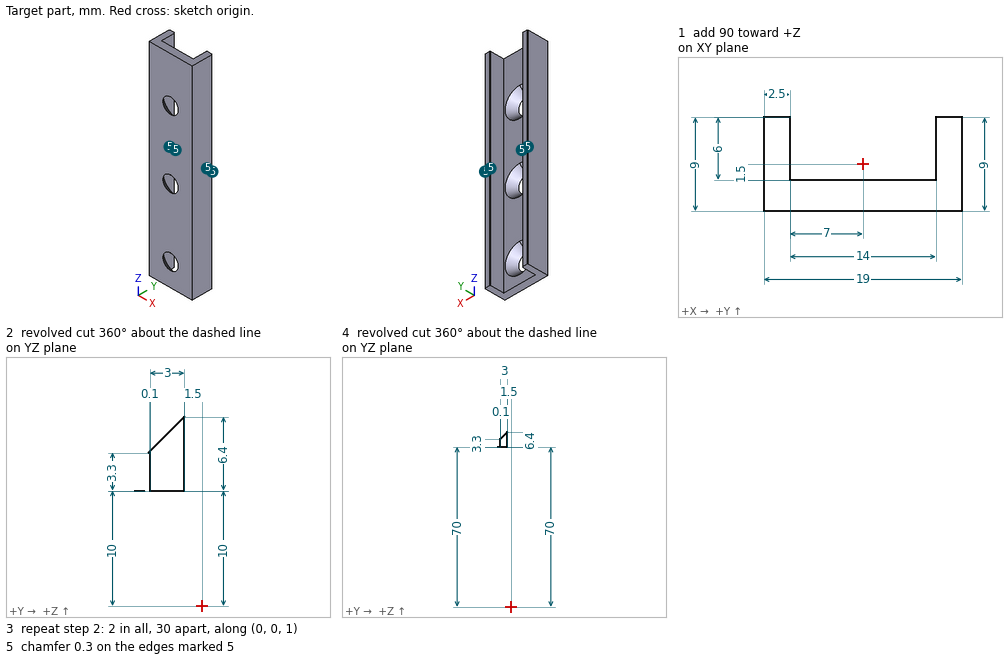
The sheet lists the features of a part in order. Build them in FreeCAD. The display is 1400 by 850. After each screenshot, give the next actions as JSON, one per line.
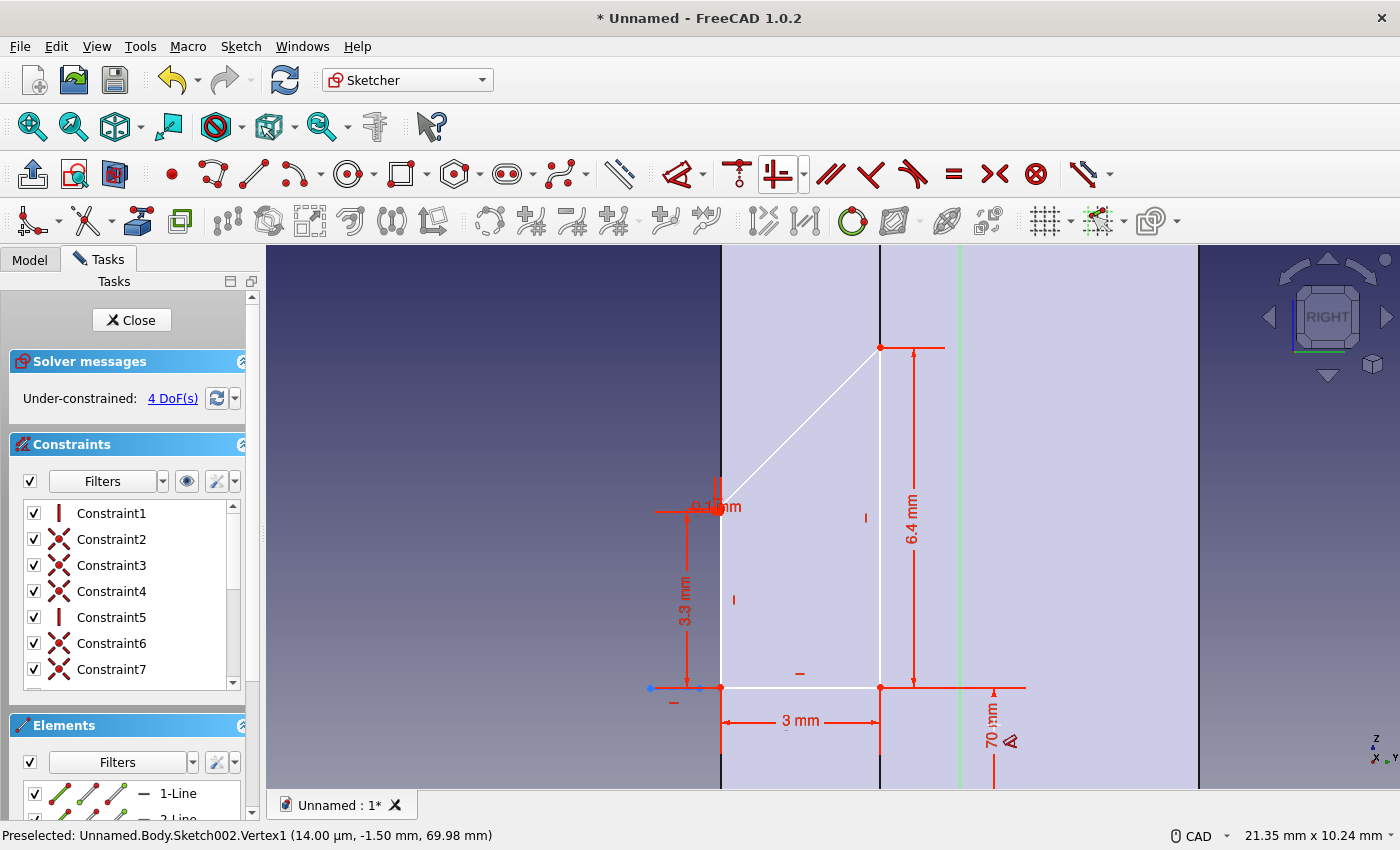
{"action": "left_click", "coordinate": [699, 689]}
{"action": "left_click", "coordinate": [994, 700]}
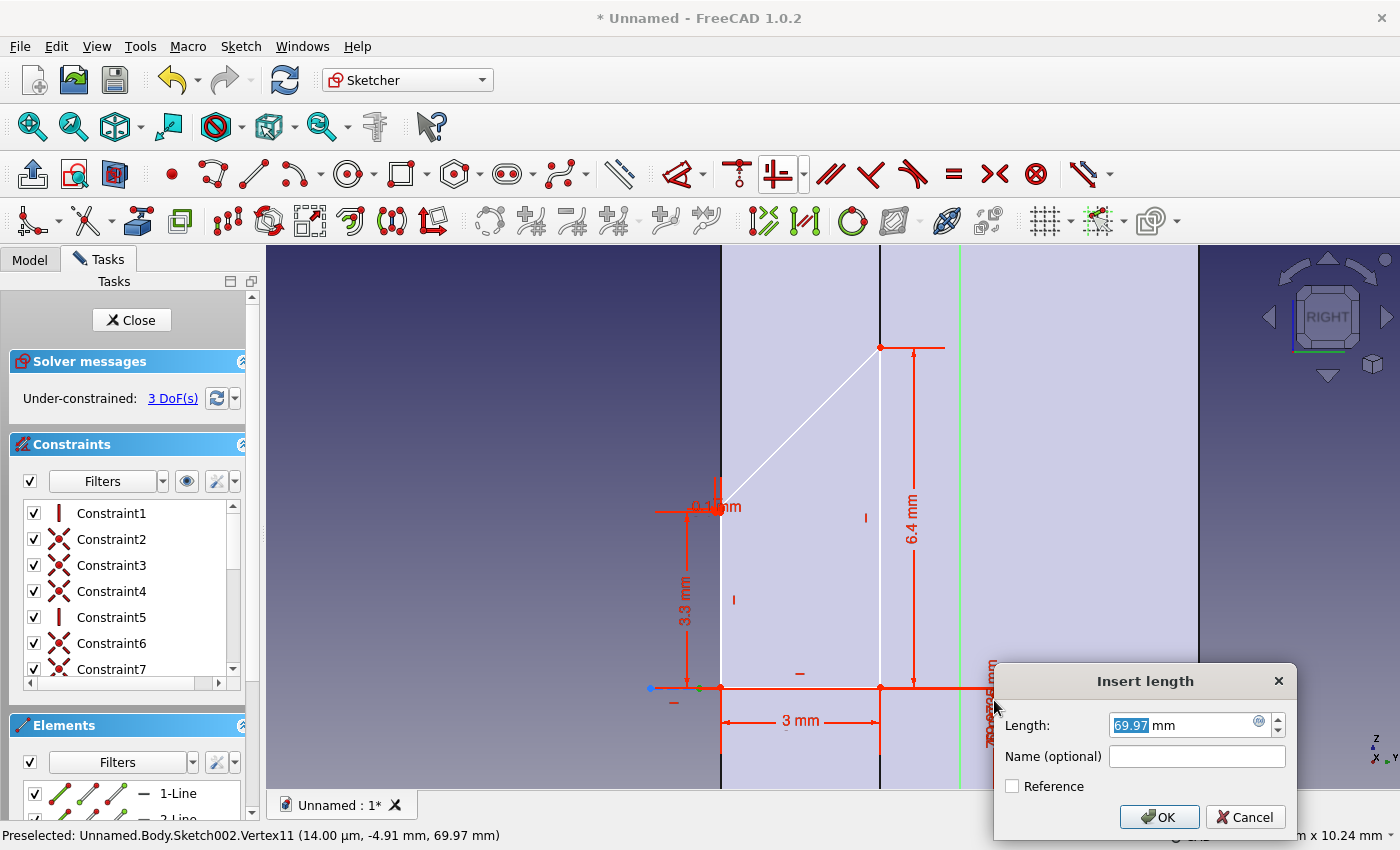
{"action": "type", "text": "70"}
{"action": "key", "text": "Return"}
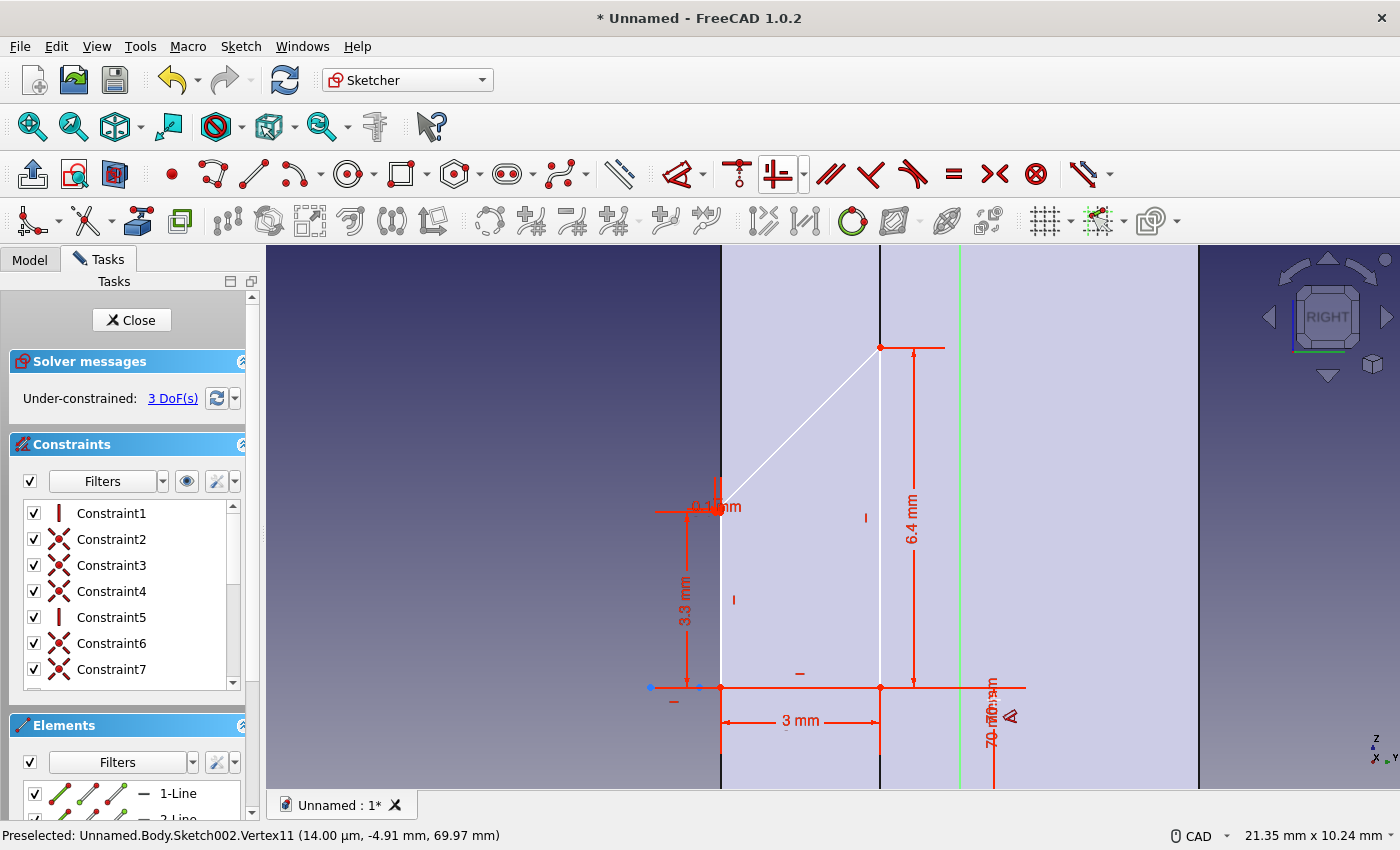
{"action": "left_click", "coordinate": [880, 688]}
{"action": "left_click", "coordinate": [920, 654]}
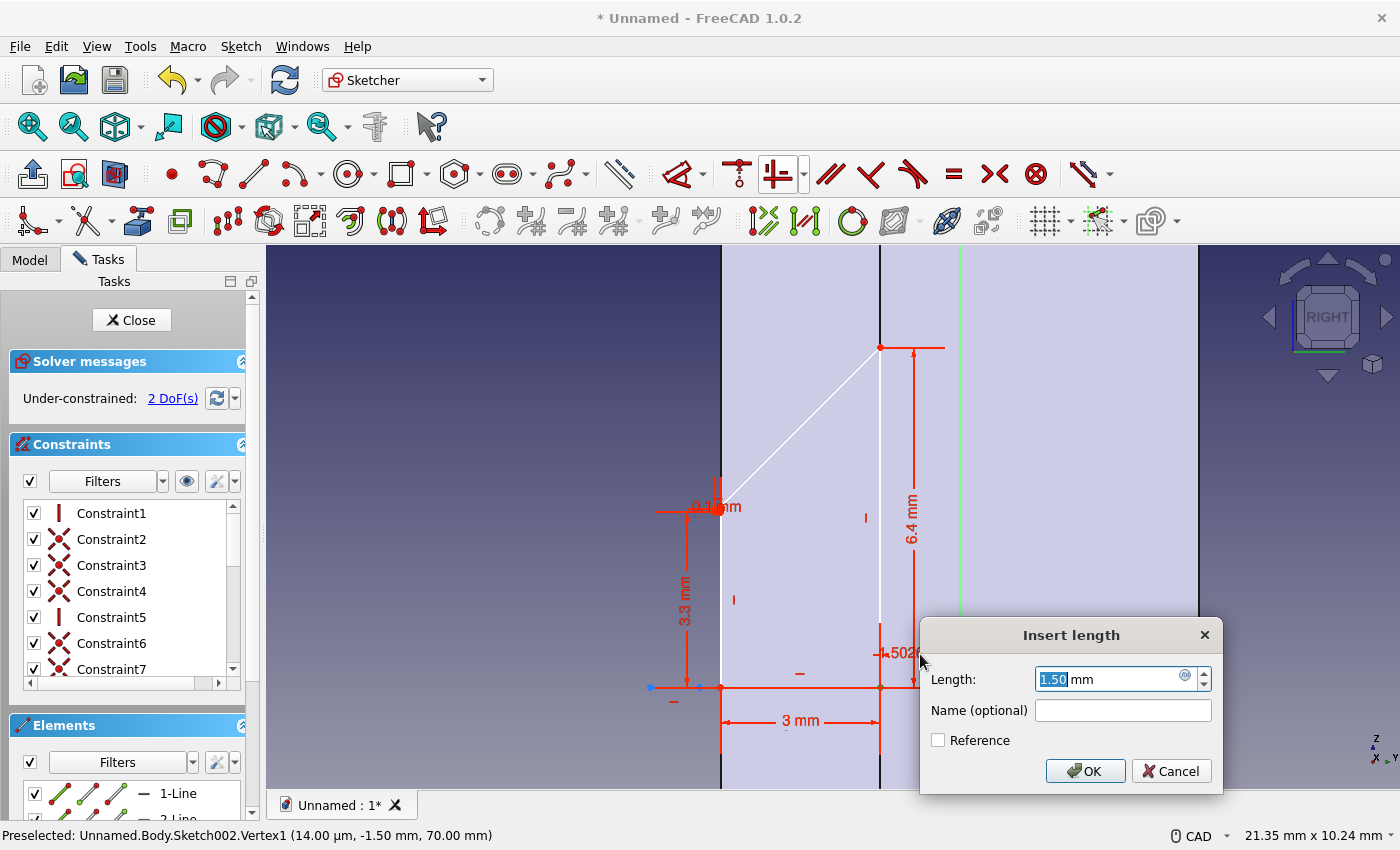
{"action": "type", "text": "1.5"}
{"action": "key", "text": "Return"}
{"action": "key", "text": "Escape"}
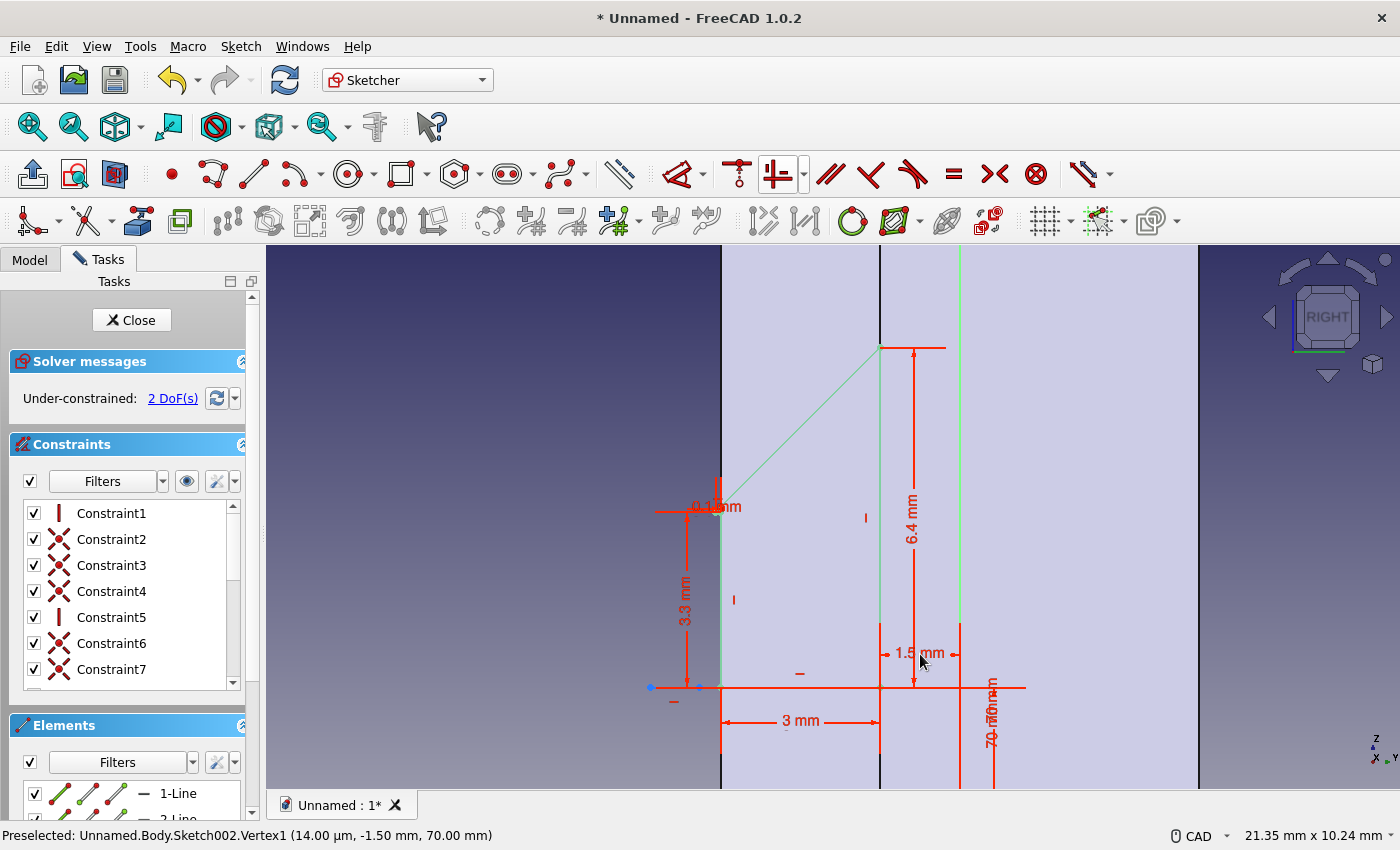
{"action": "left_click", "coordinate": [132, 320]}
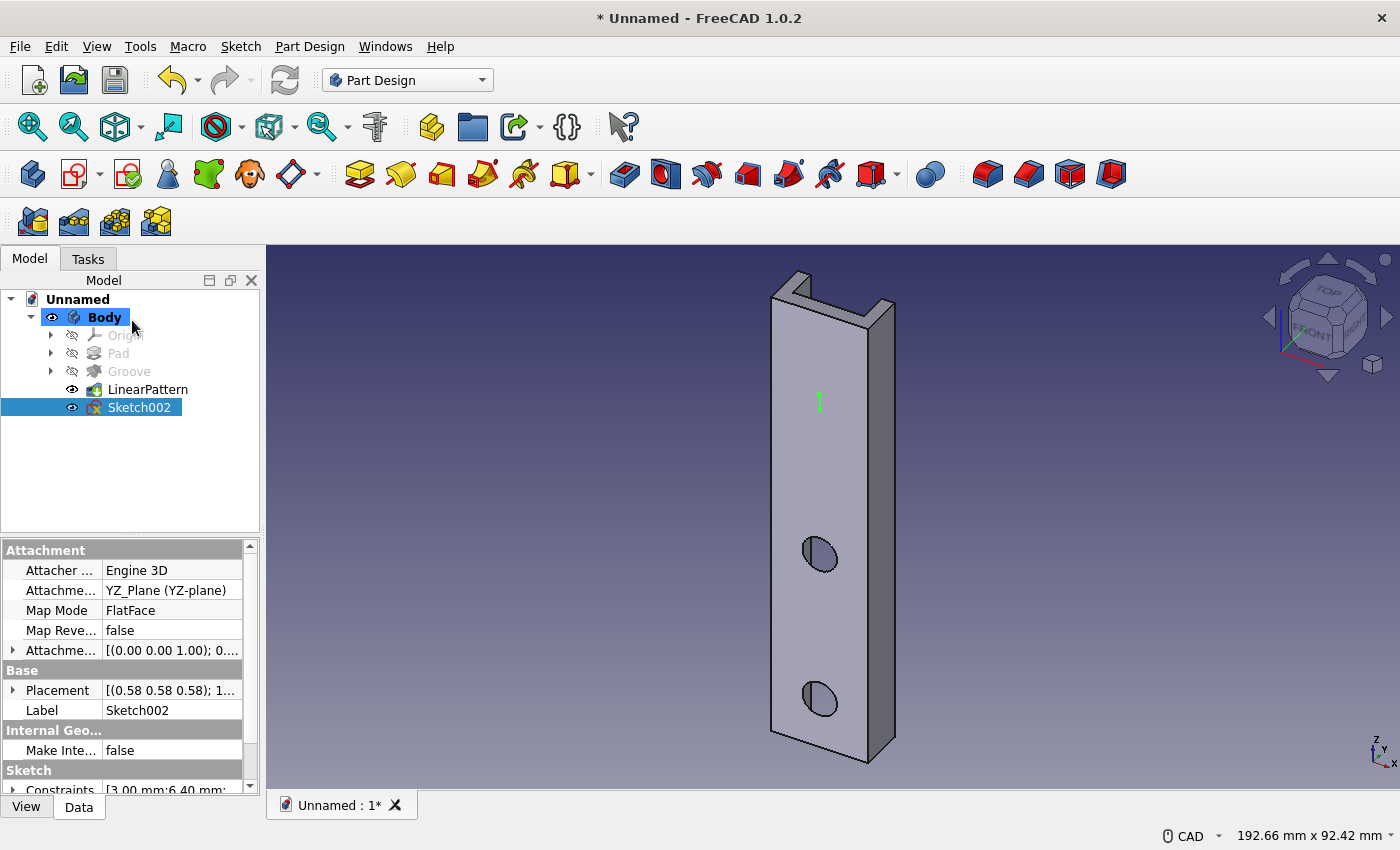
{"action": "left_click", "coordinate": [707, 174]}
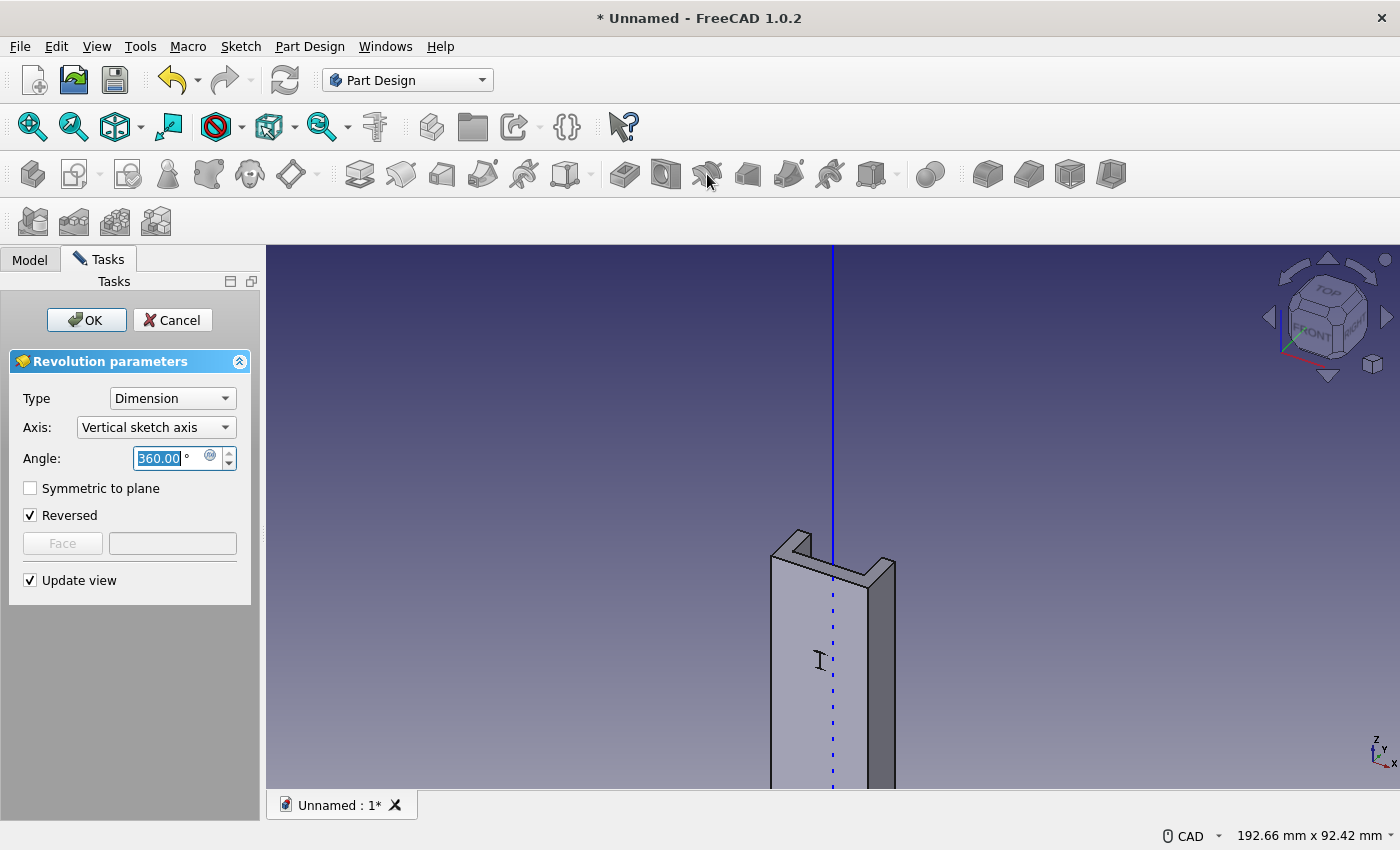
{"action": "left_click", "coordinate": [157, 428]}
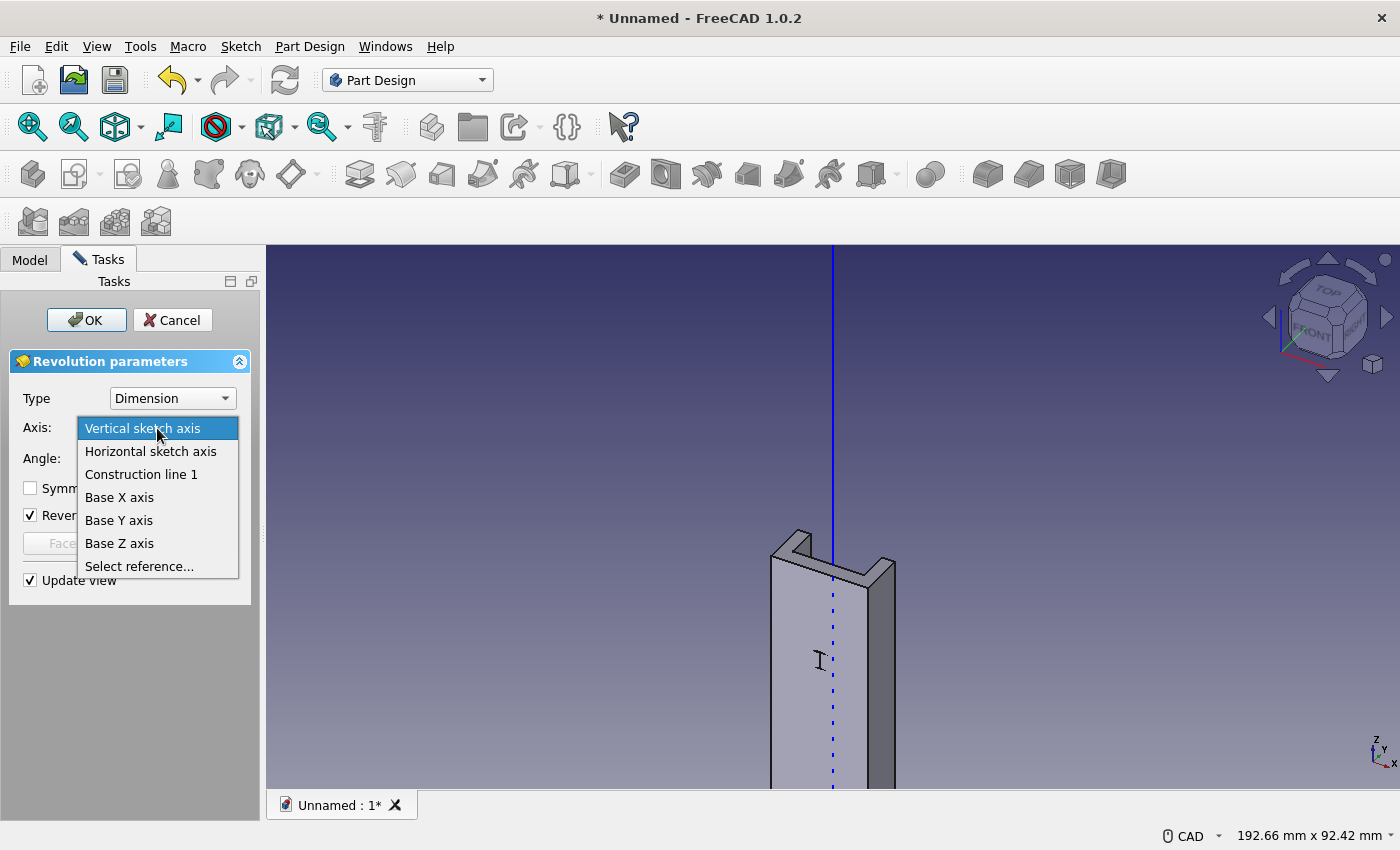
{"action": "left_click", "coordinate": [156, 474]}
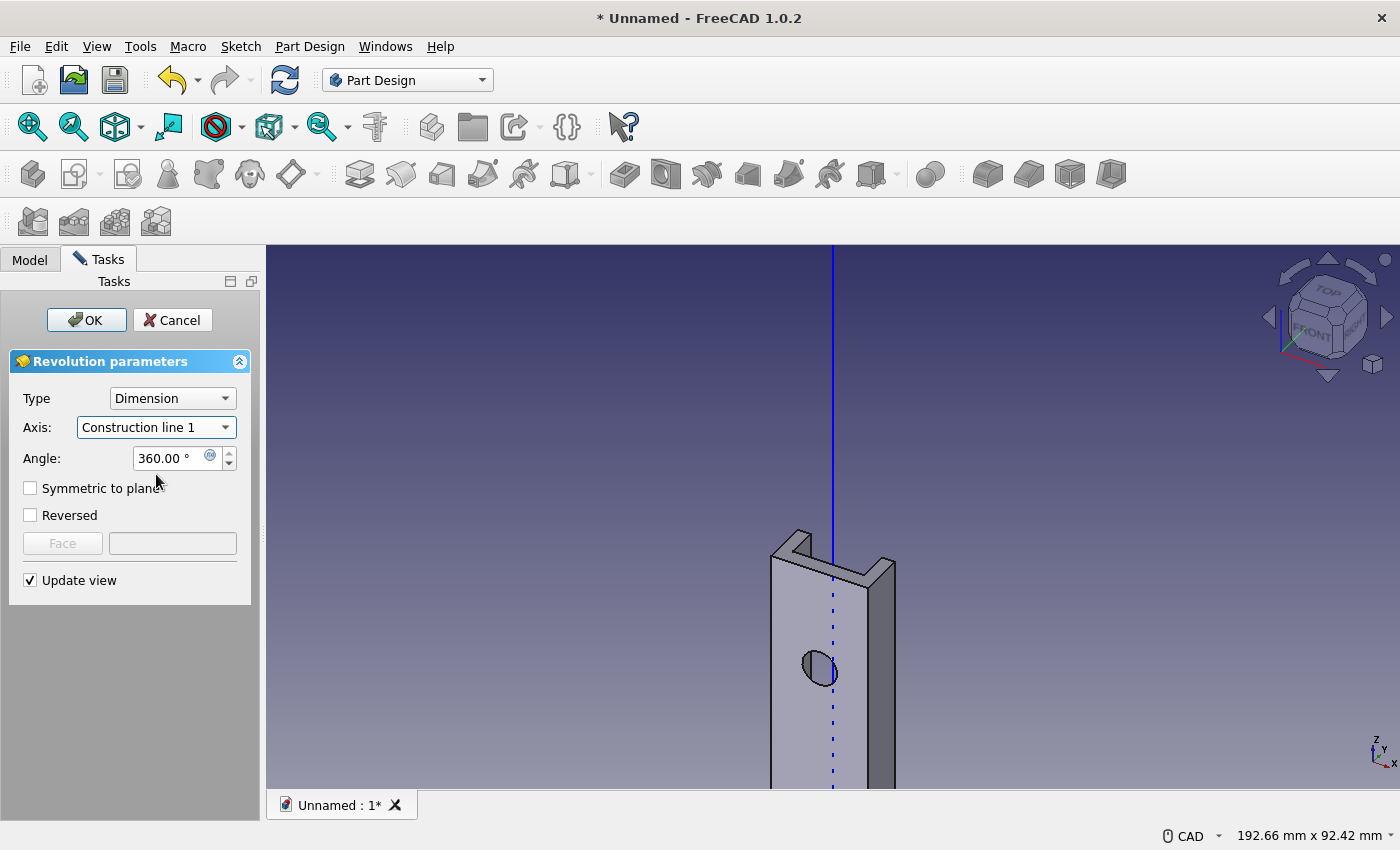
{"action": "left_click", "coordinate": [87, 320]}